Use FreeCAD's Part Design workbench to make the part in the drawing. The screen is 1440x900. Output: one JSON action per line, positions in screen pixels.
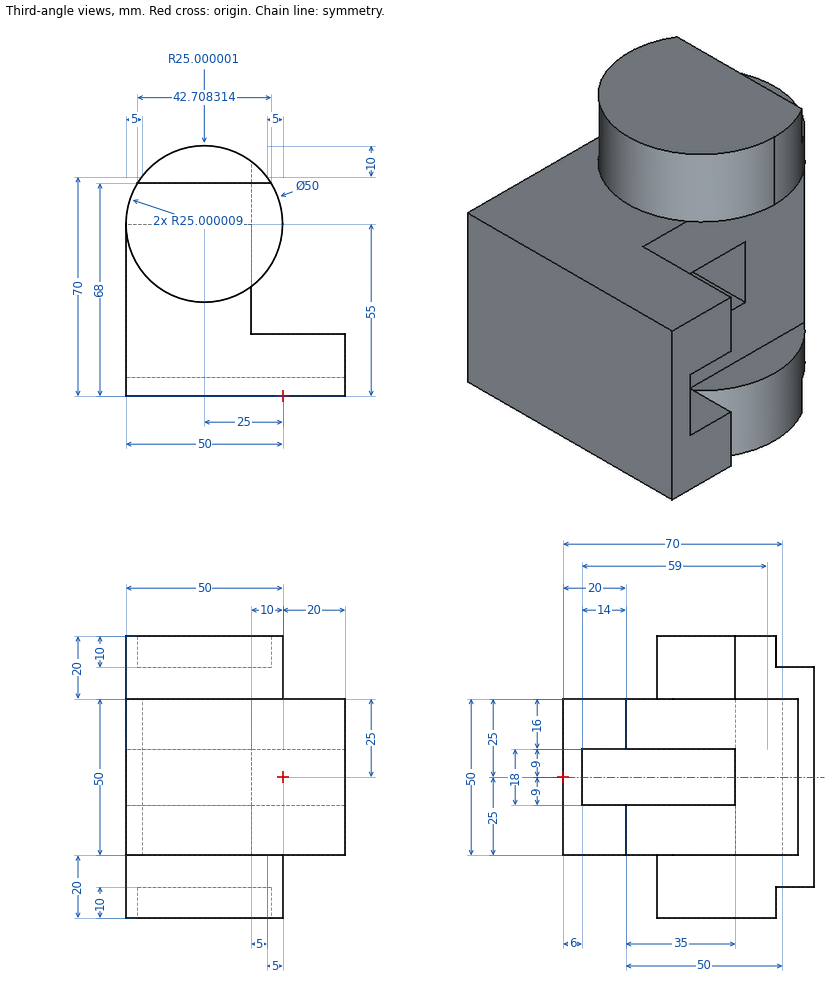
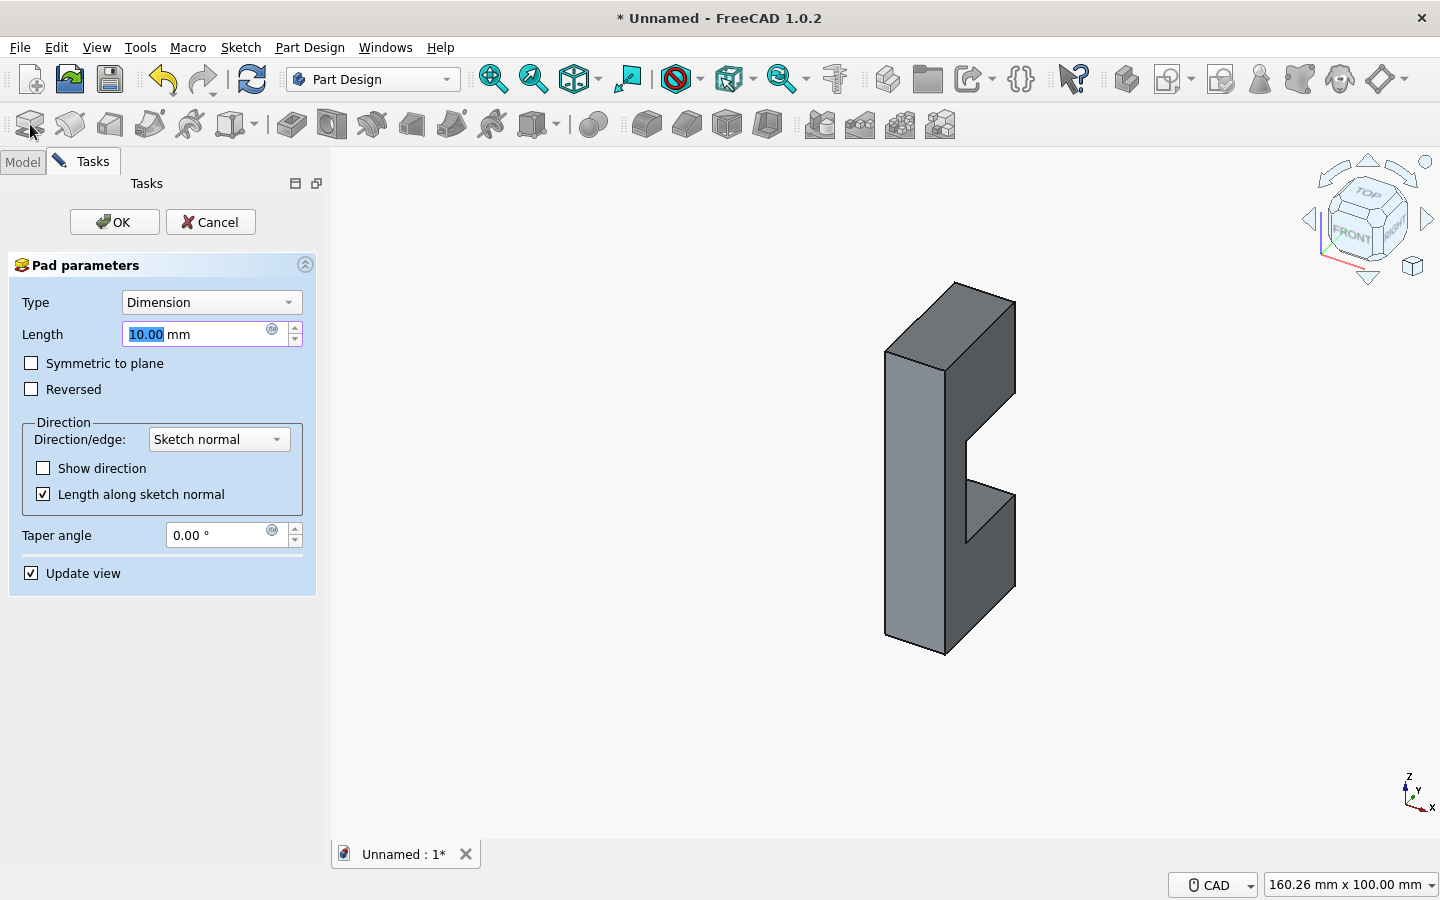
{"action": "type", "text": "20"}
{"action": "key", "text": "Tab"}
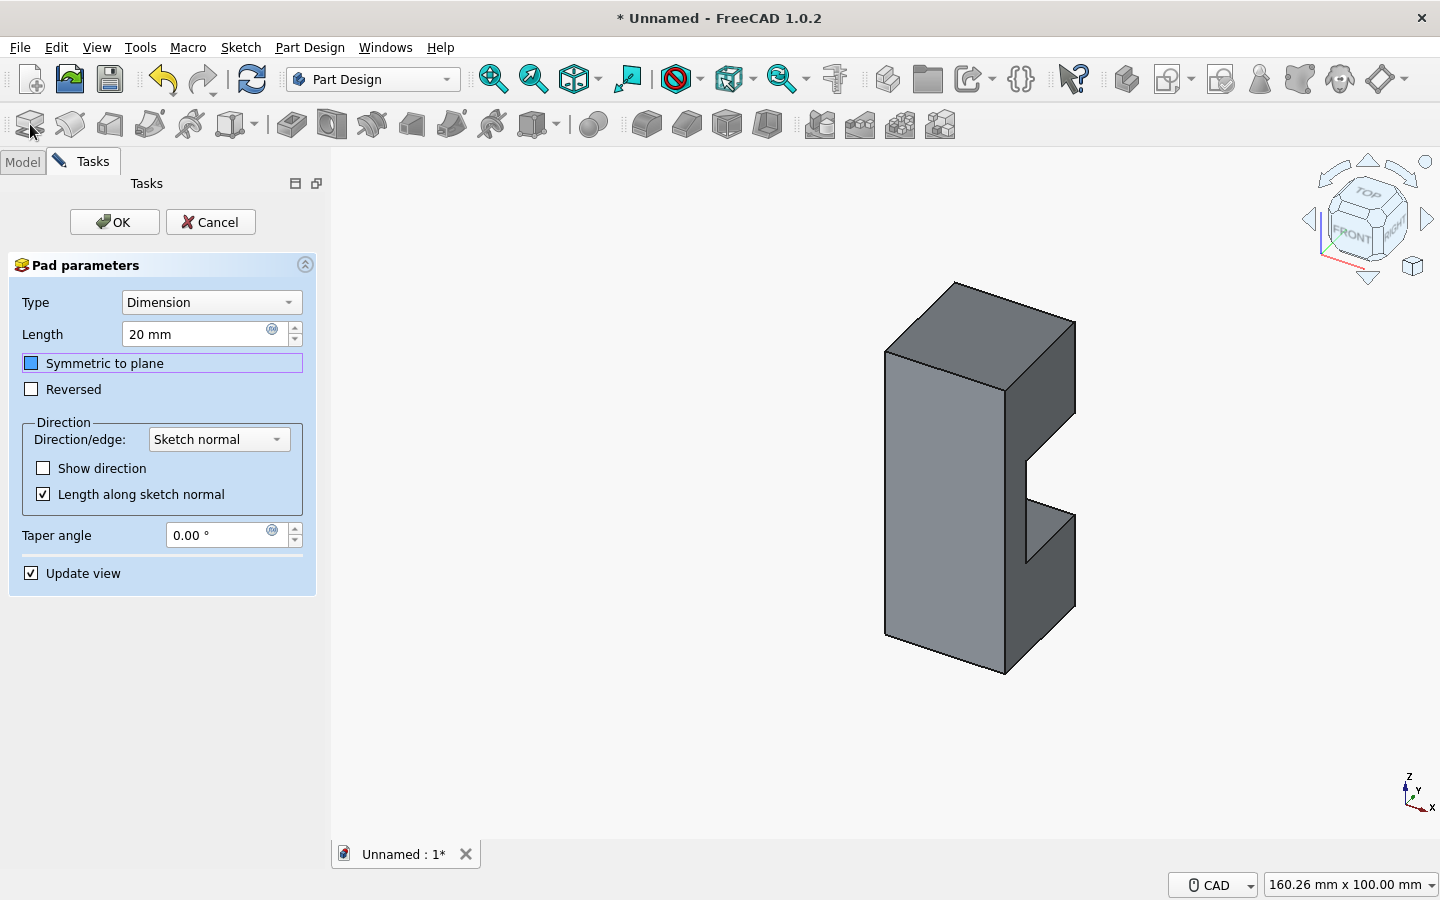
{"action": "left_click", "coordinate": [115, 222]}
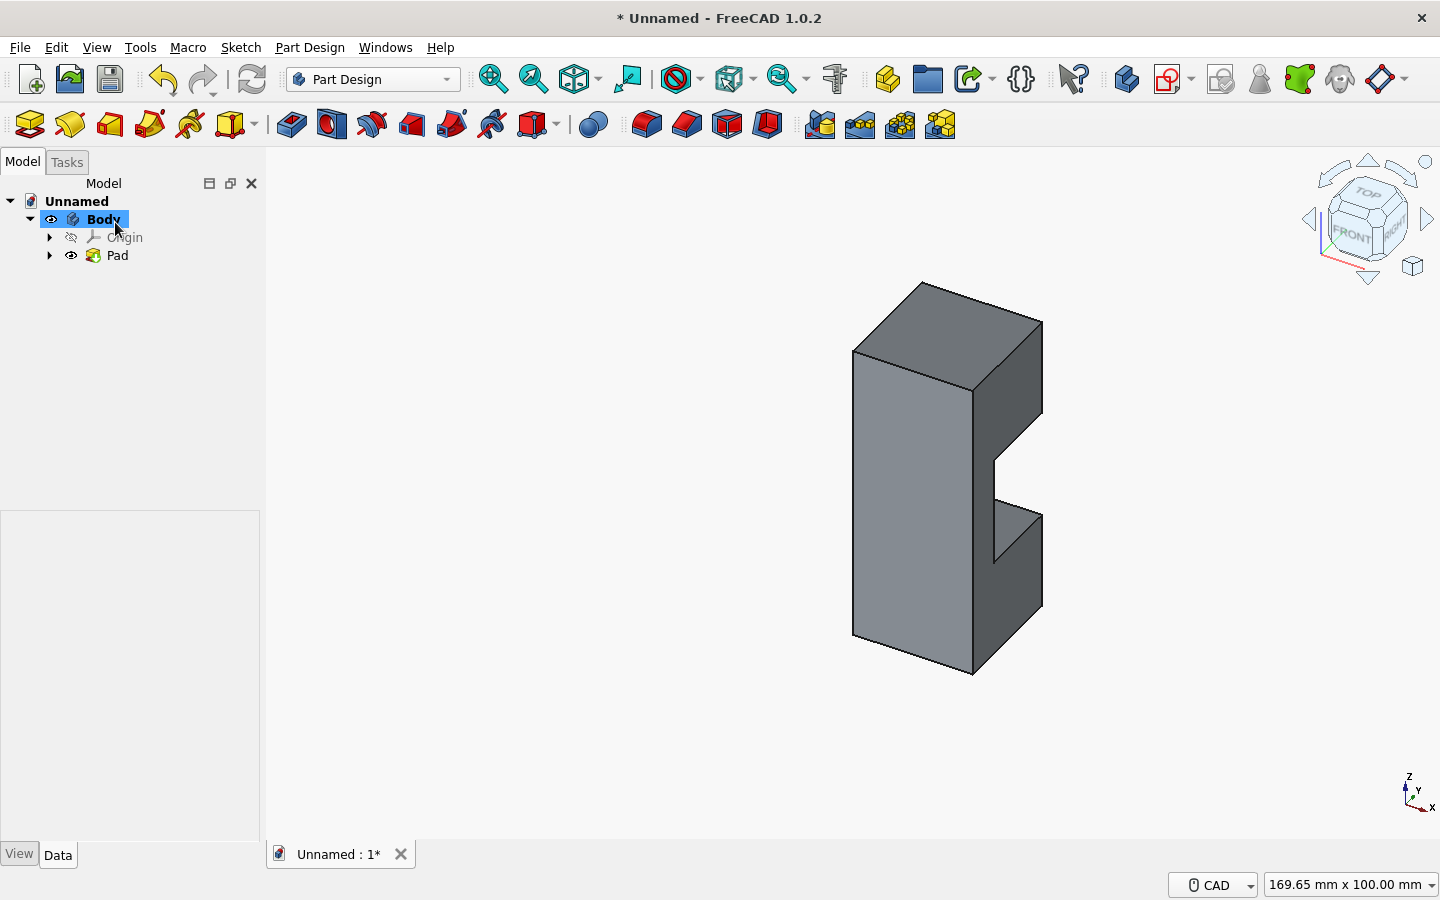
{"action": "key", "text": "6"}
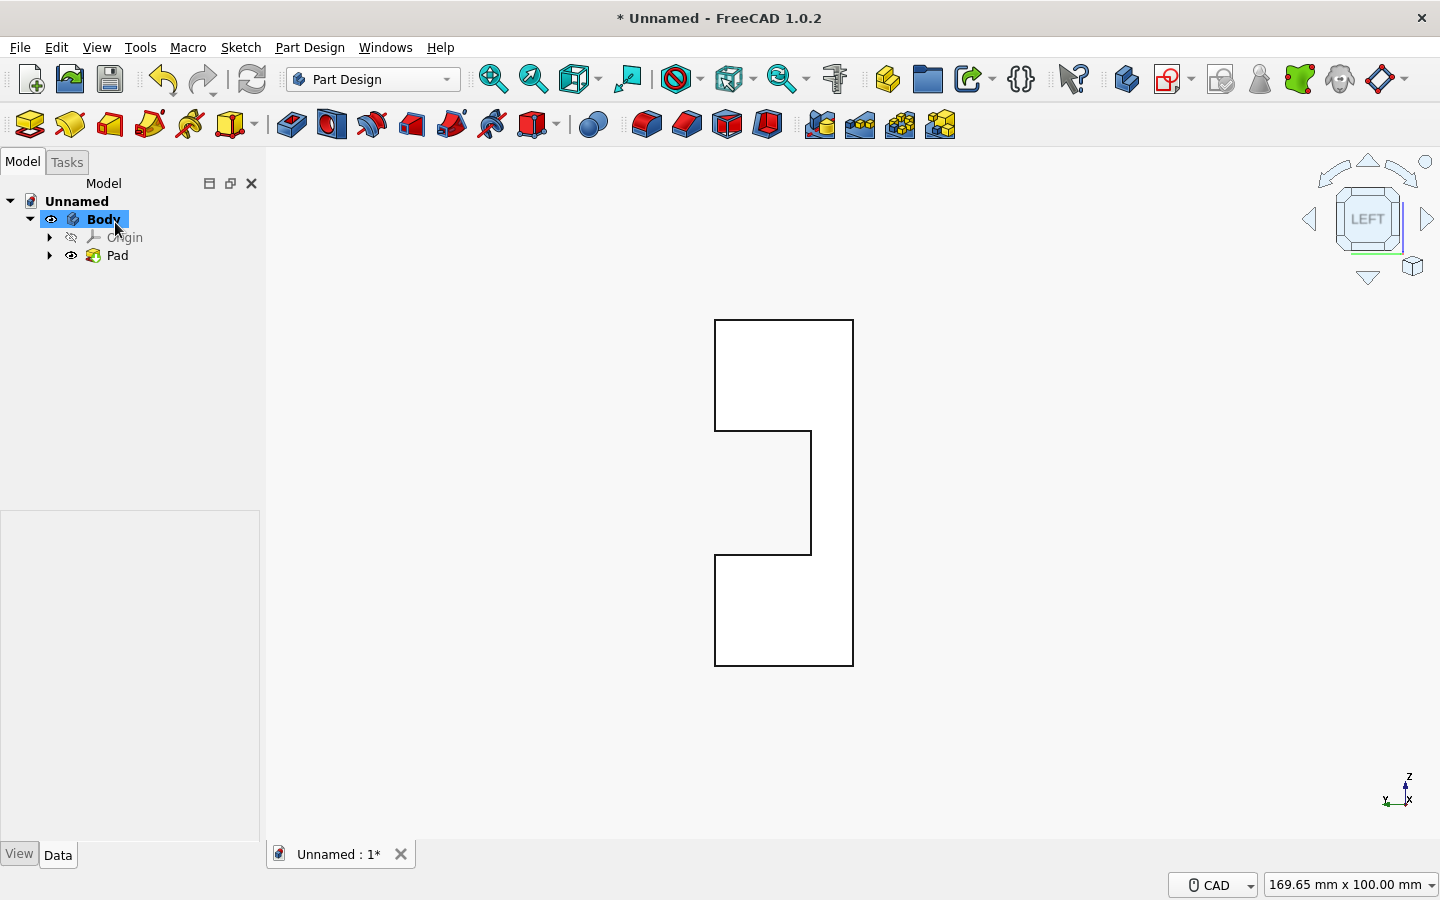
{"action": "left_click", "coordinate": [784, 591]}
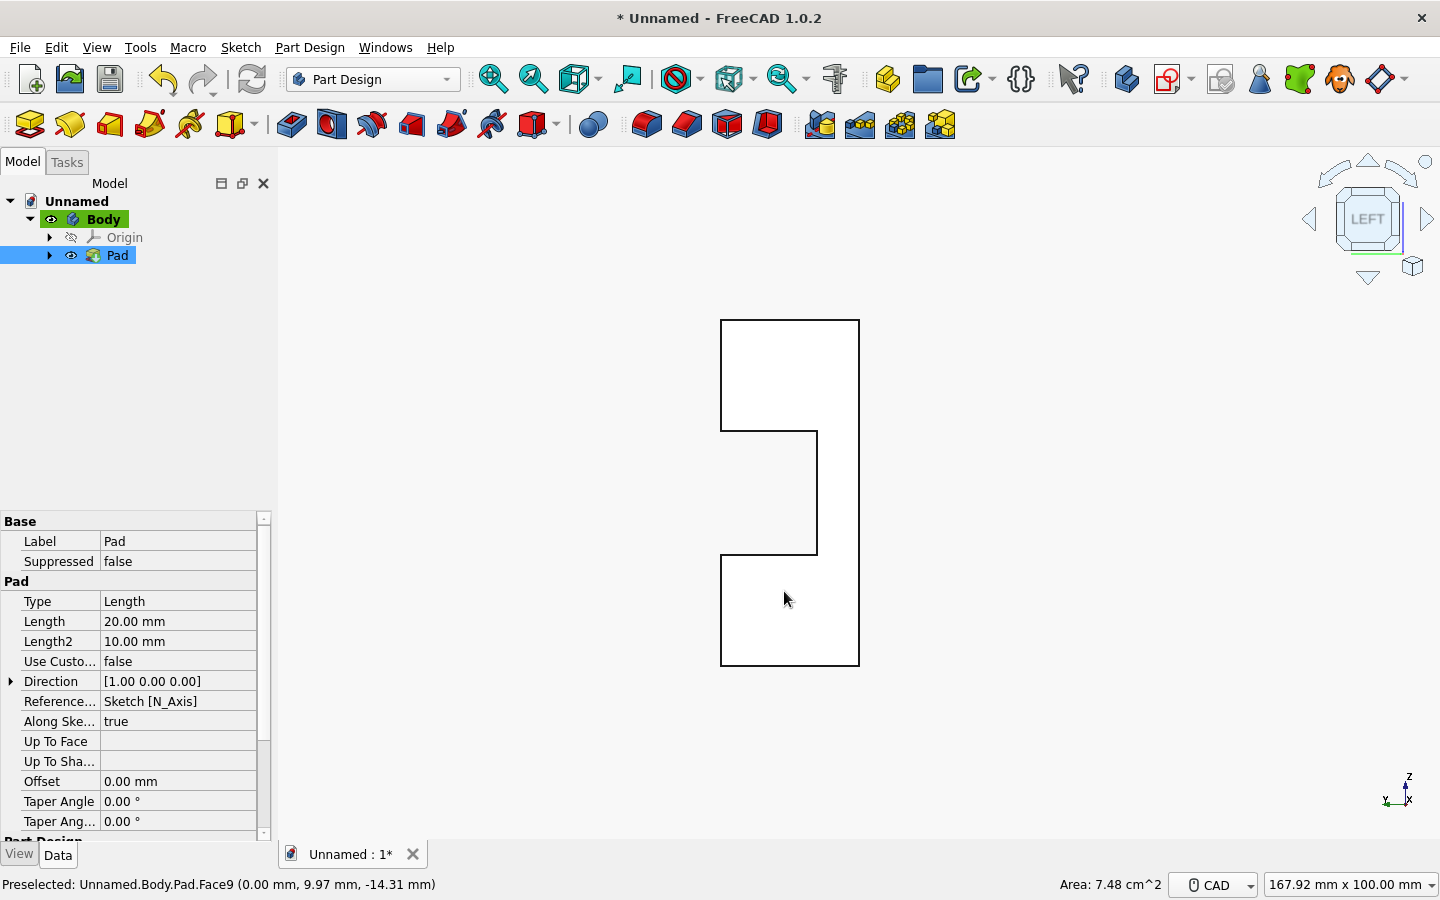
{"action": "left_click", "coordinate": [1168, 80]}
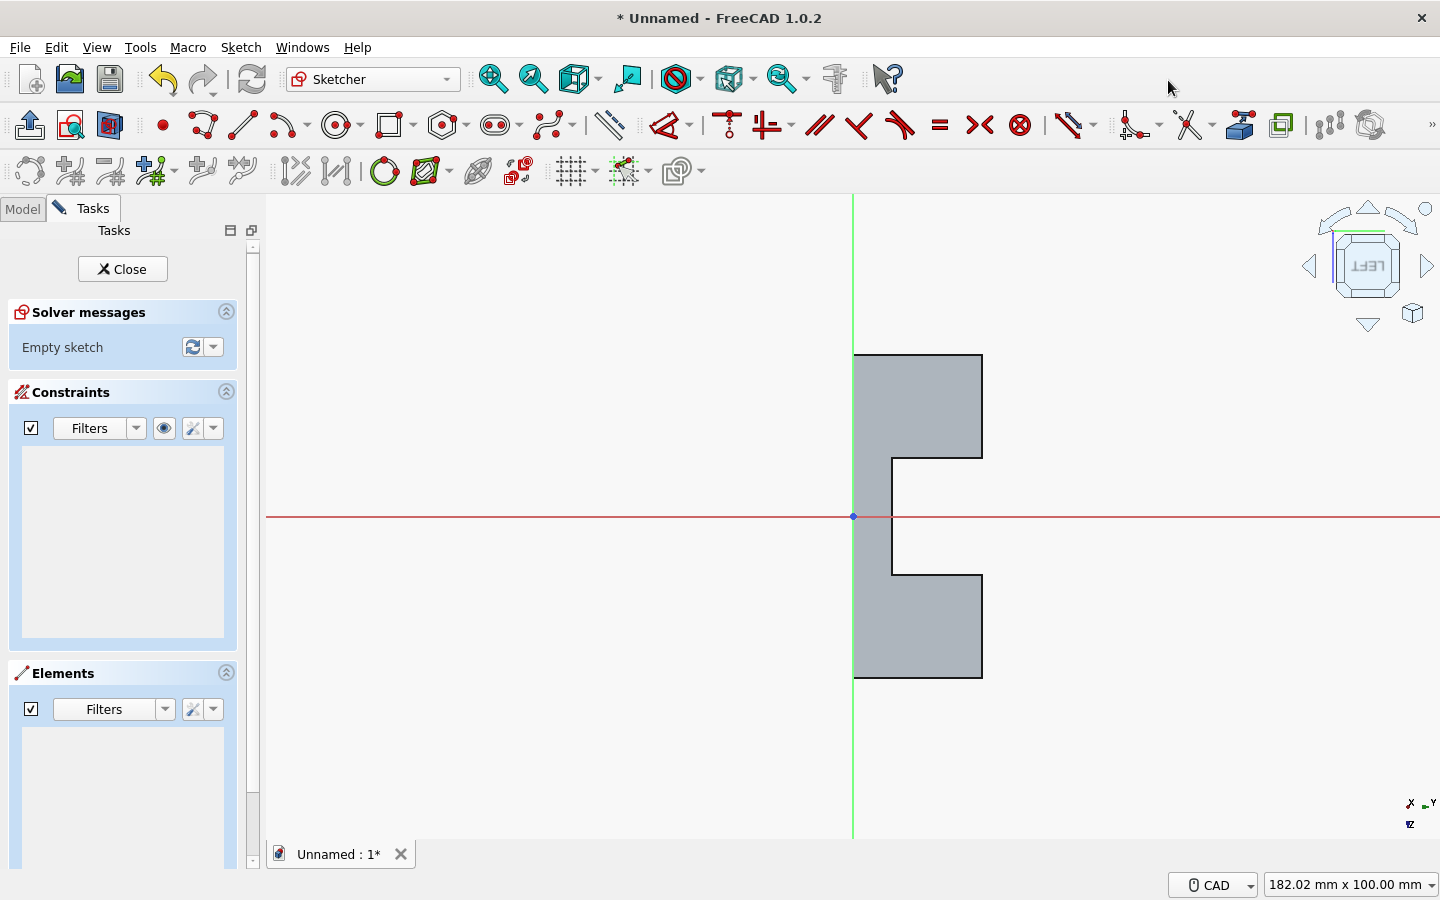
{"action": "scroll", "coordinate": [294, 516], "scroll_direction": "down", "scroll_amount": 1}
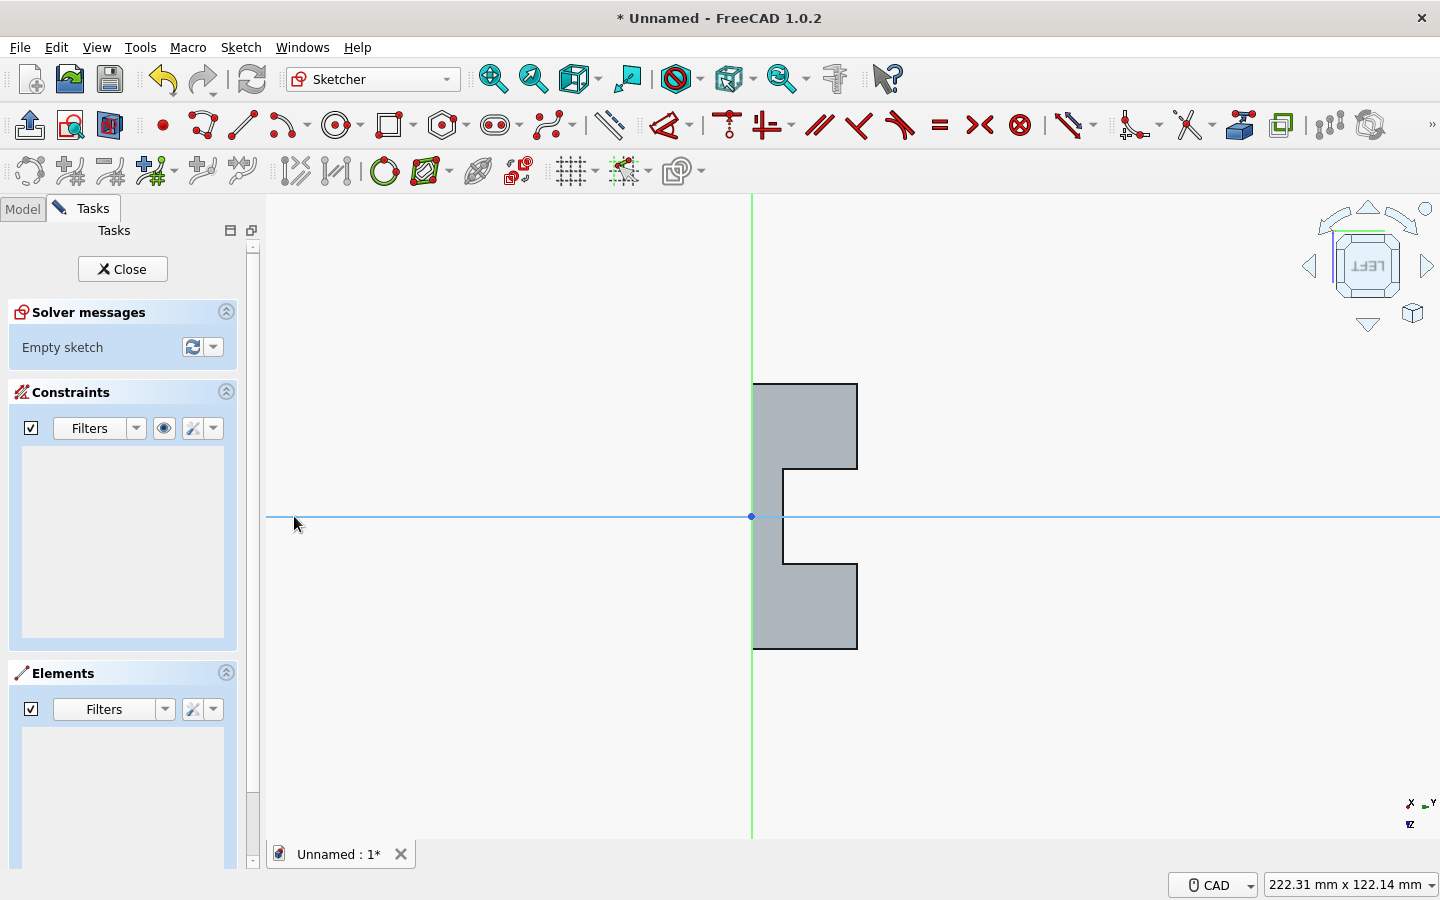
{"action": "scroll", "coordinate": [1246, 517], "scroll_direction": "up", "scroll_amount": 2}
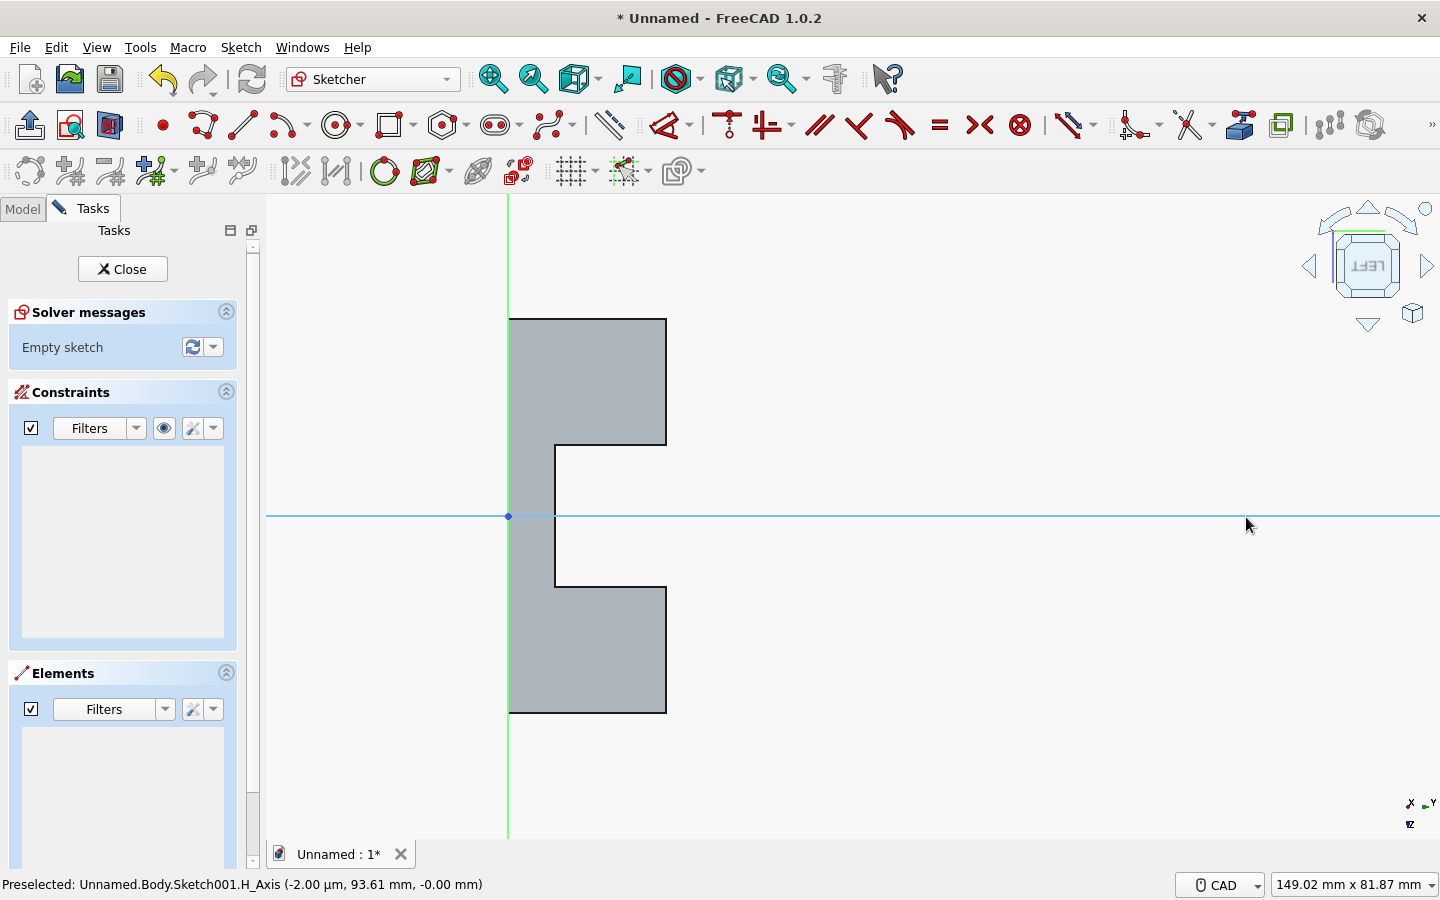
{"action": "key", "text": "g r"}